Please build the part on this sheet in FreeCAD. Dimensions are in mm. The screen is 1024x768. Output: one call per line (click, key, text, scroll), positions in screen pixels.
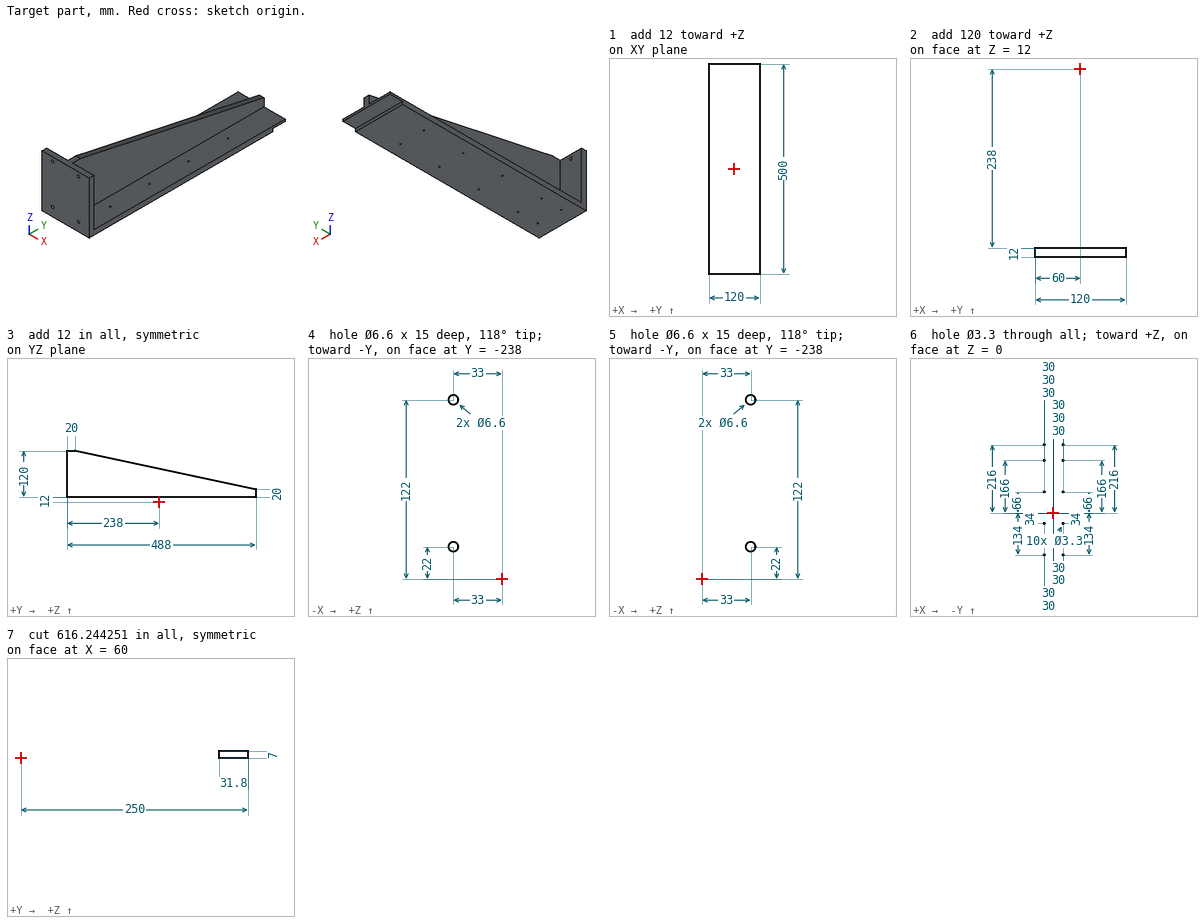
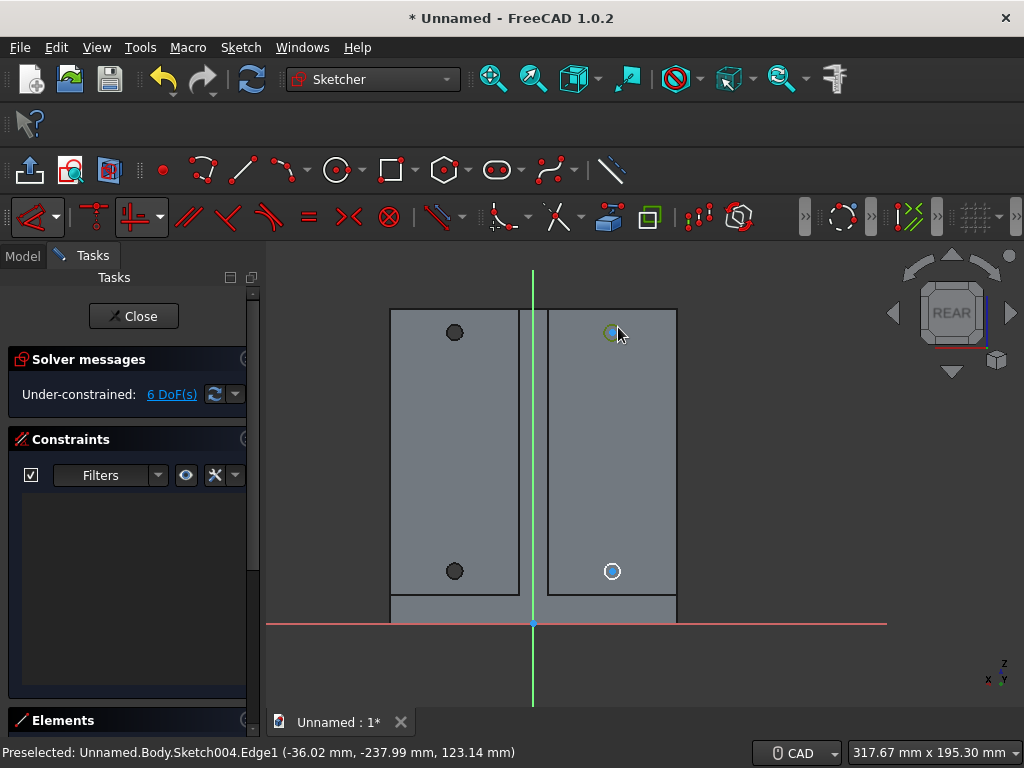
scroll(618, 566, up, 3)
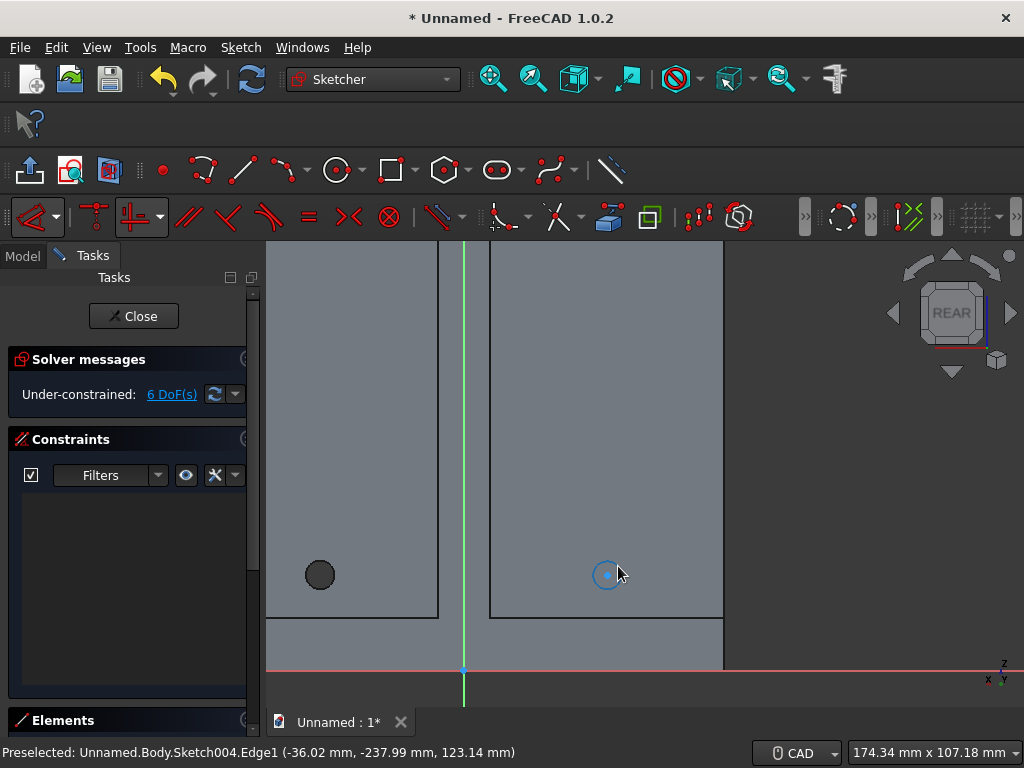
click(617, 565)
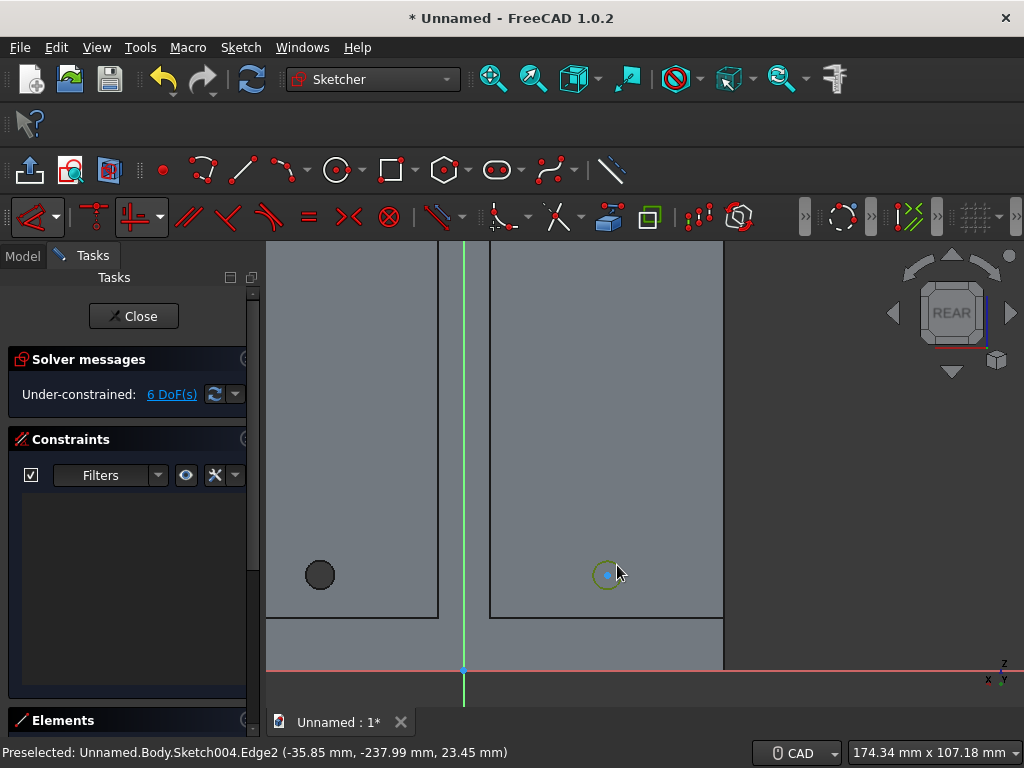
click(310, 218)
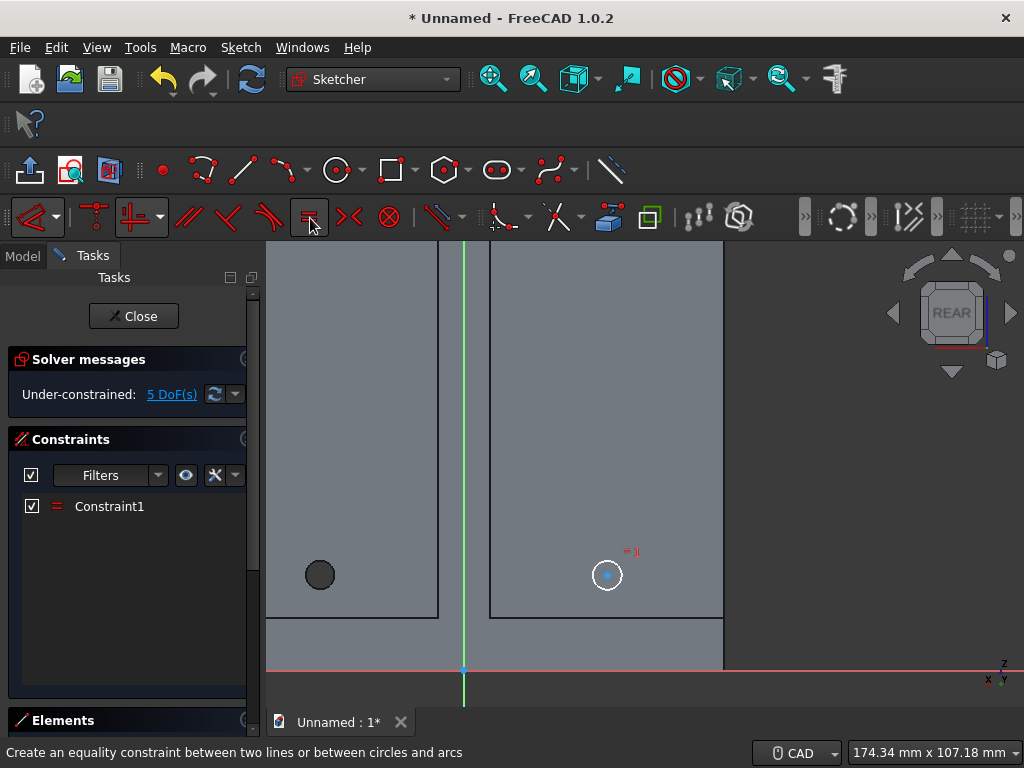
scroll(618, 566, down, 3)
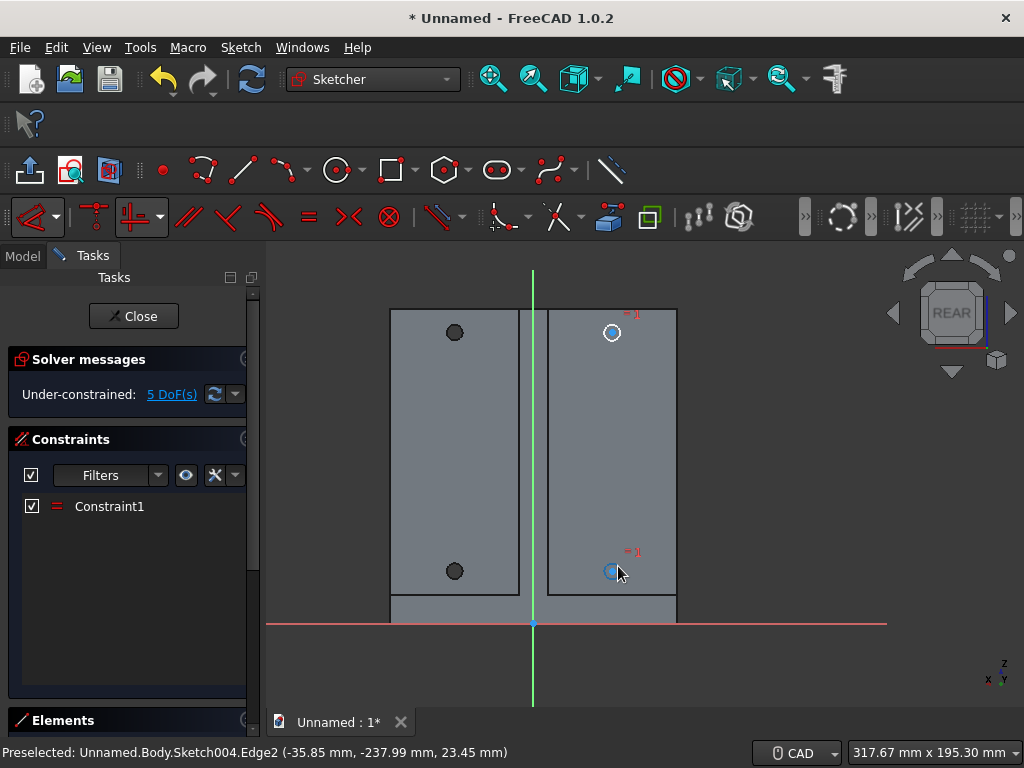
scroll(618, 327, up, 5)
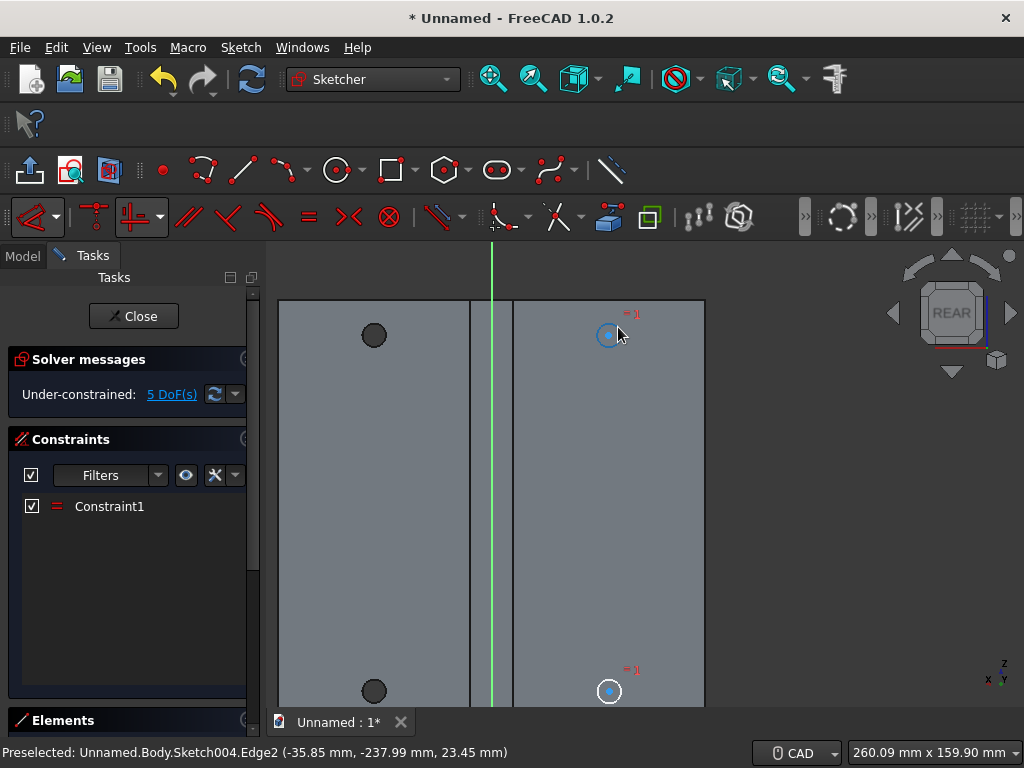
click(616, 327)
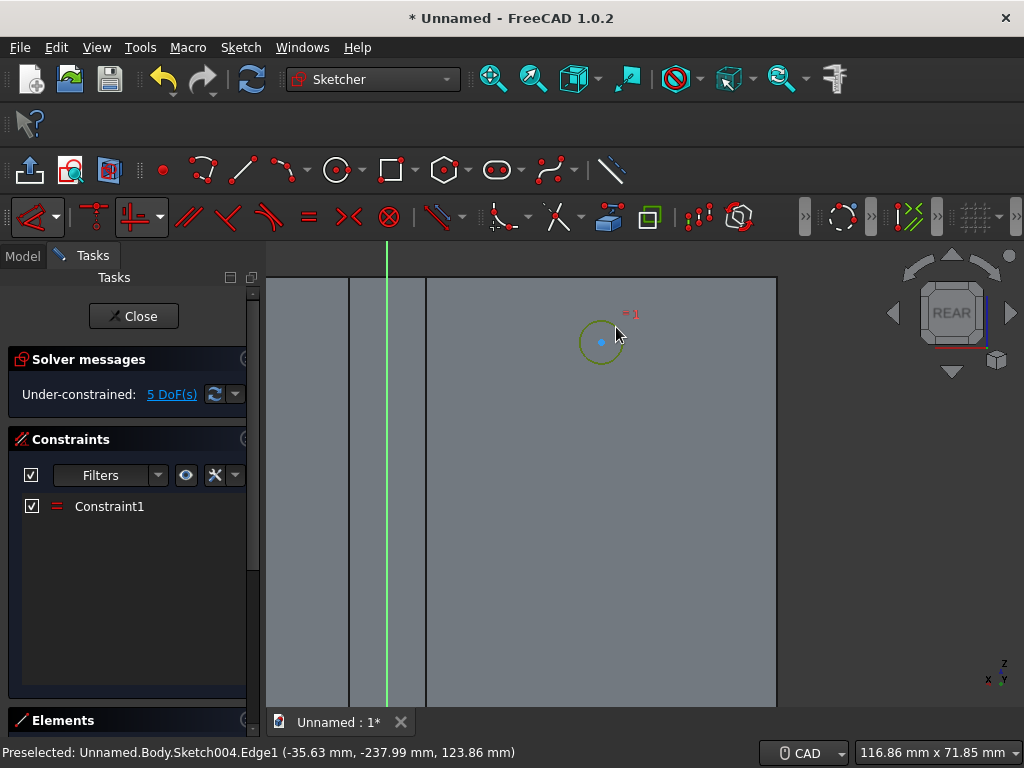
key(k)
key(o)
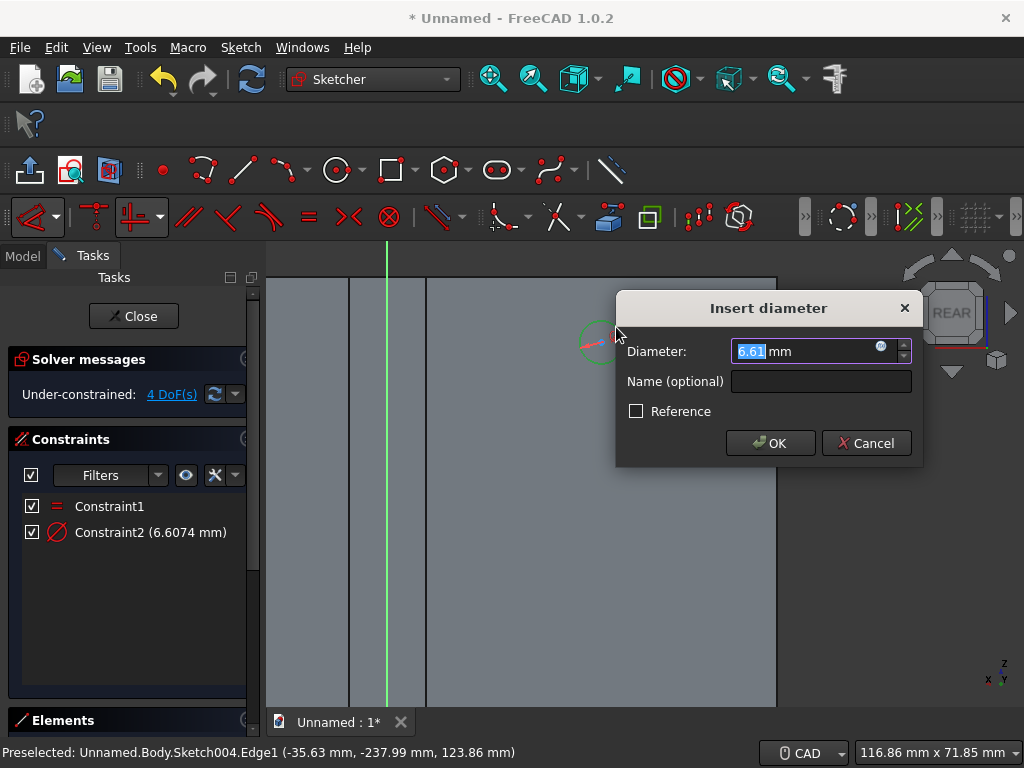
text(6.6)
key(Return)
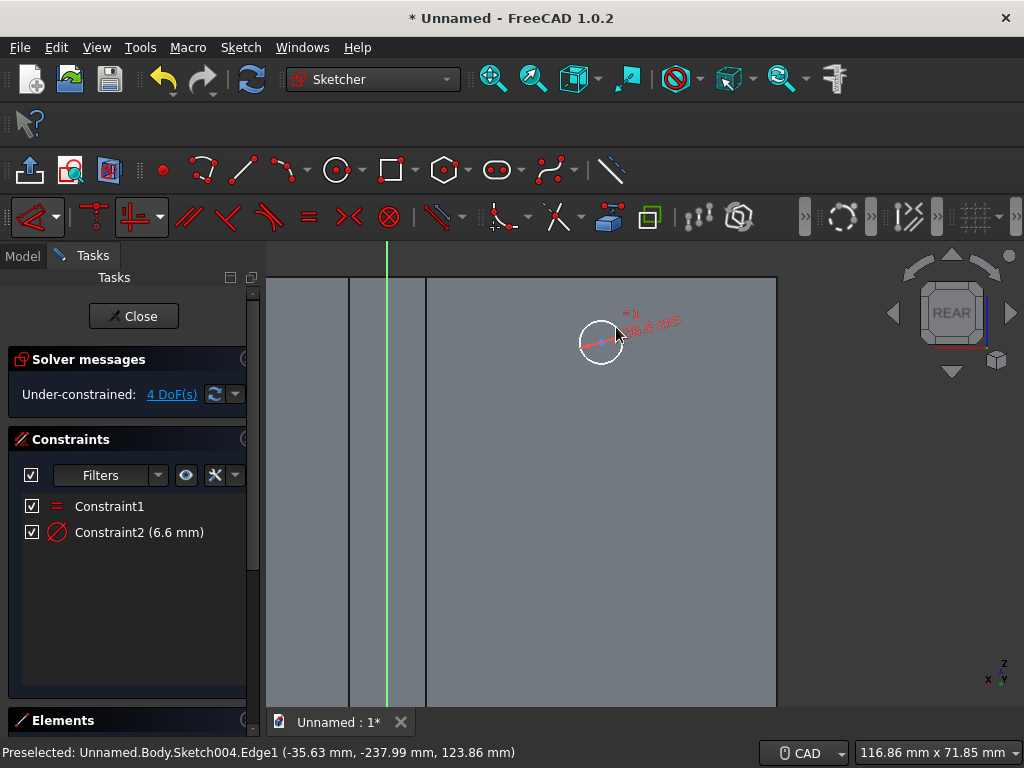
click(601, 342)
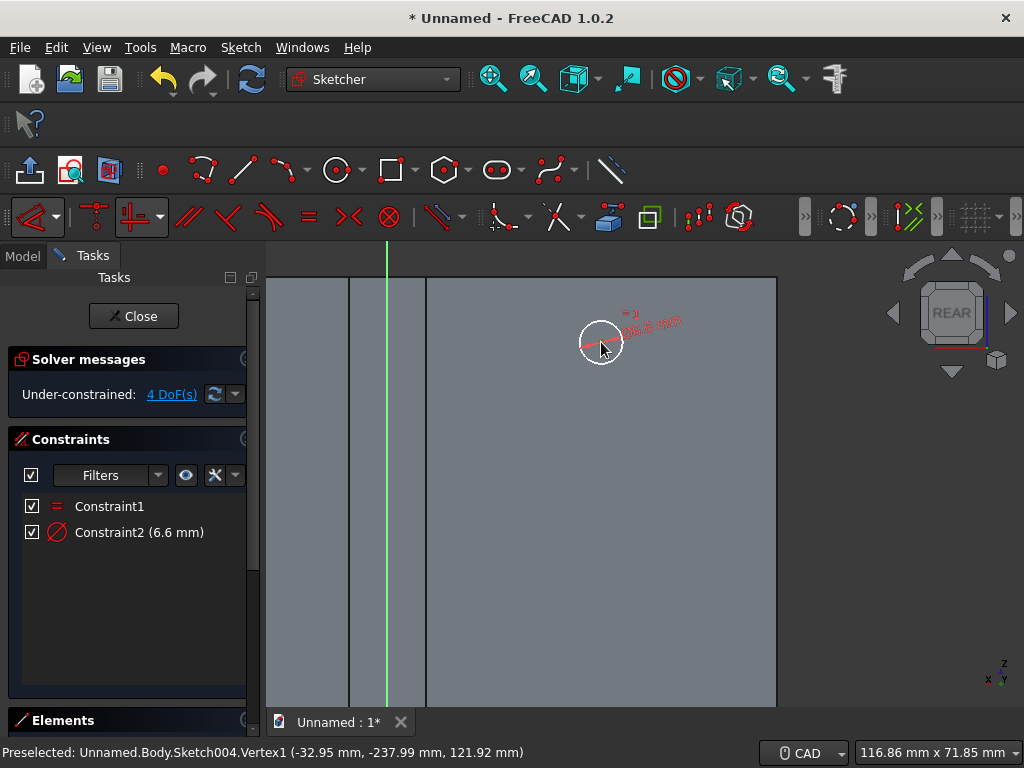
click(58, 218)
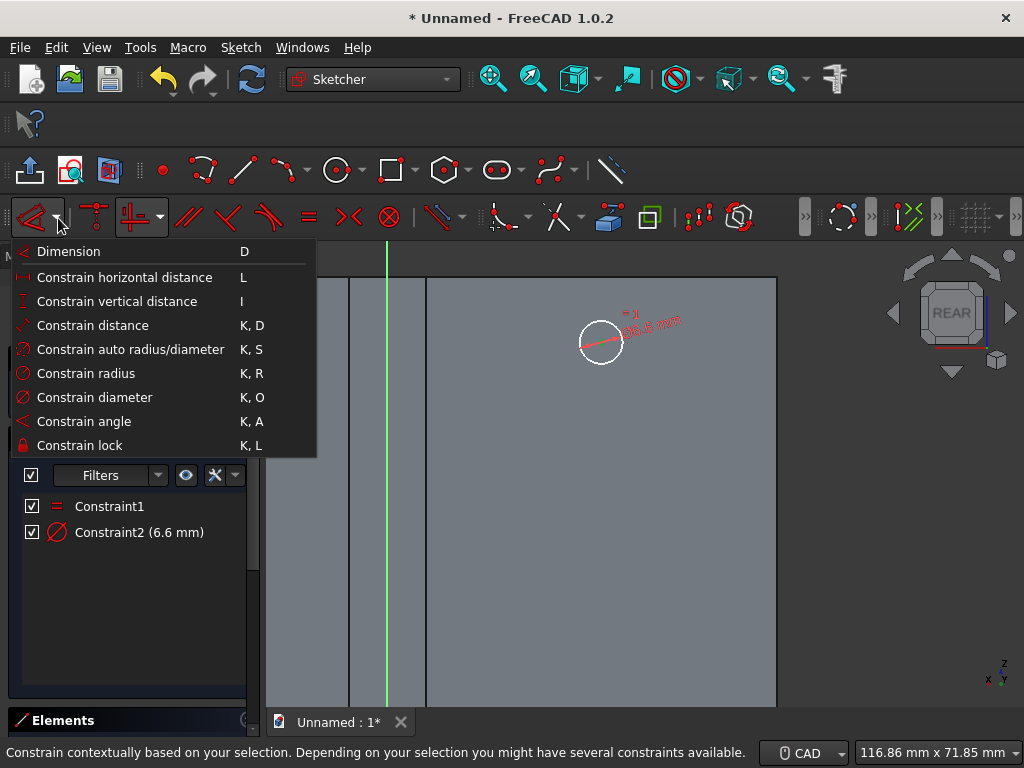
click(164, 277)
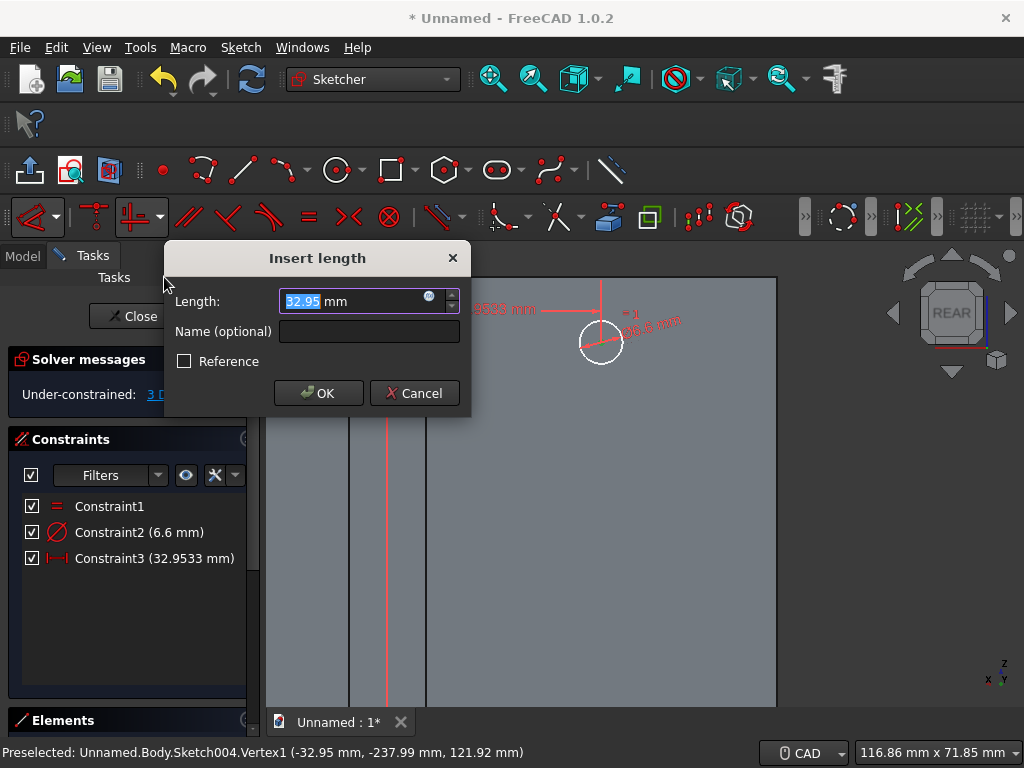
text(33)
key(Return)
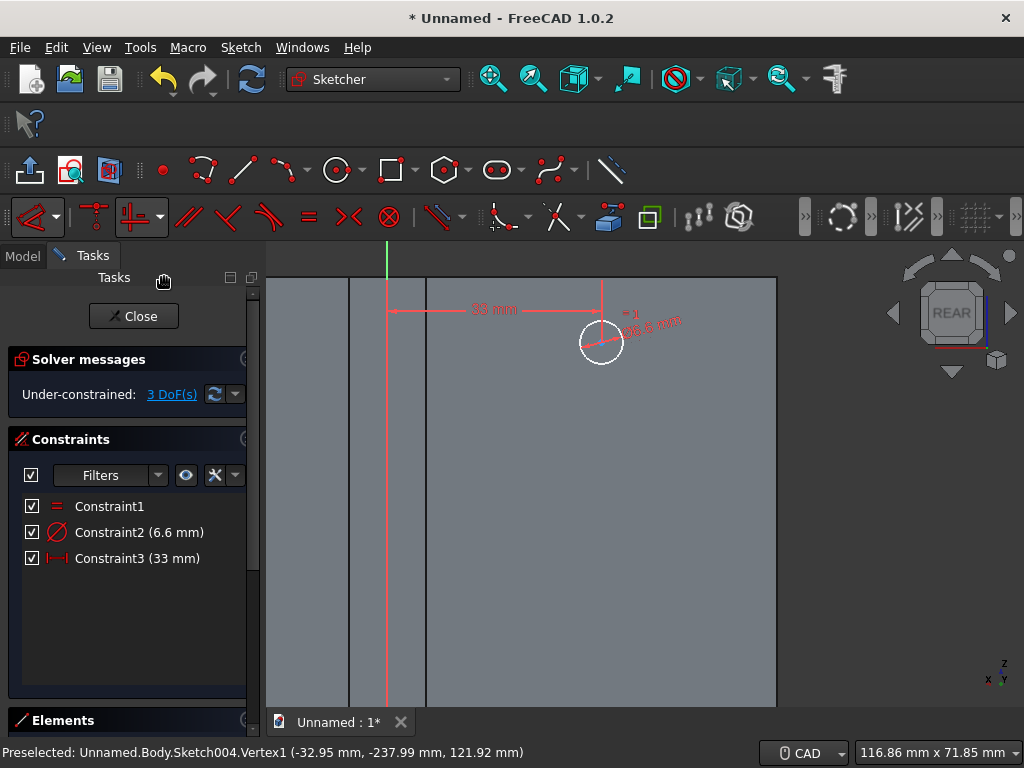
scroll(618, 327, down, 5)